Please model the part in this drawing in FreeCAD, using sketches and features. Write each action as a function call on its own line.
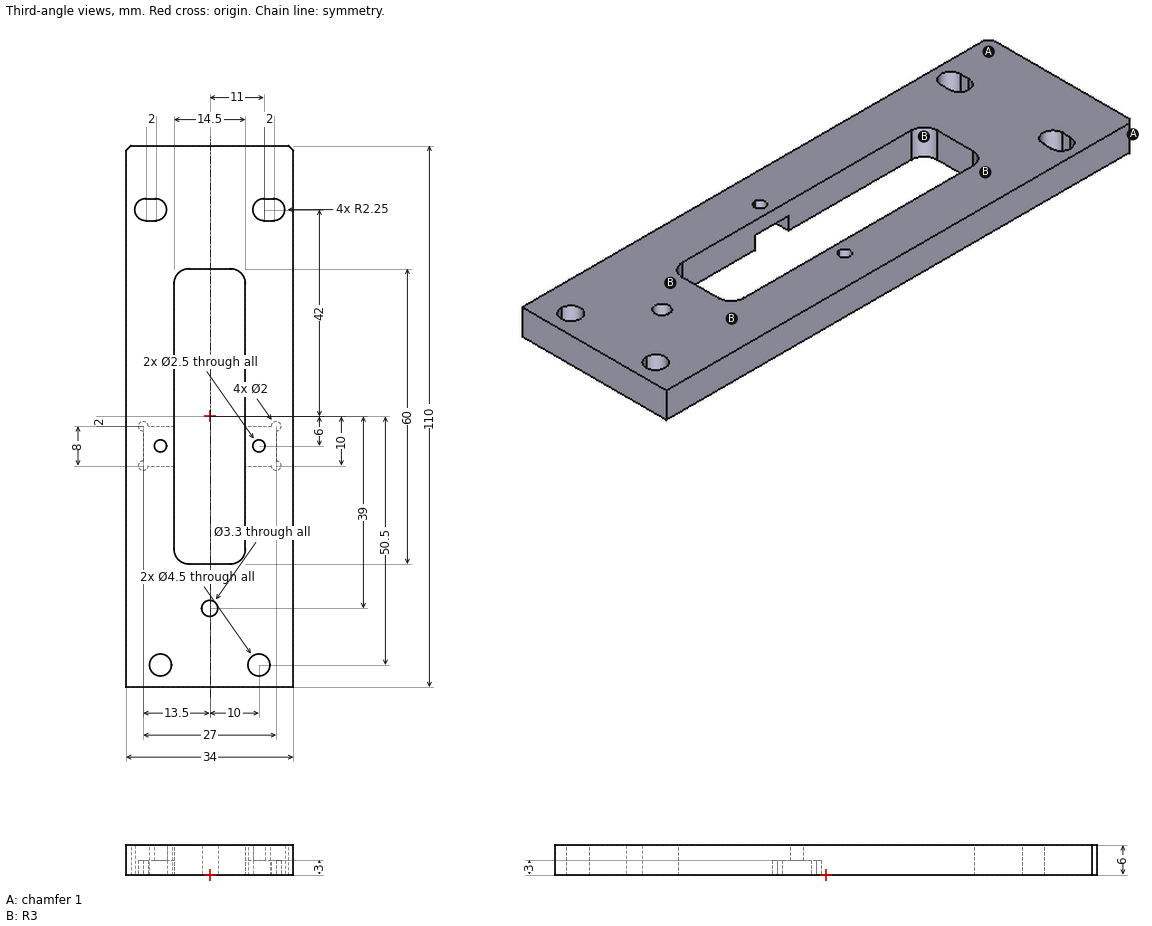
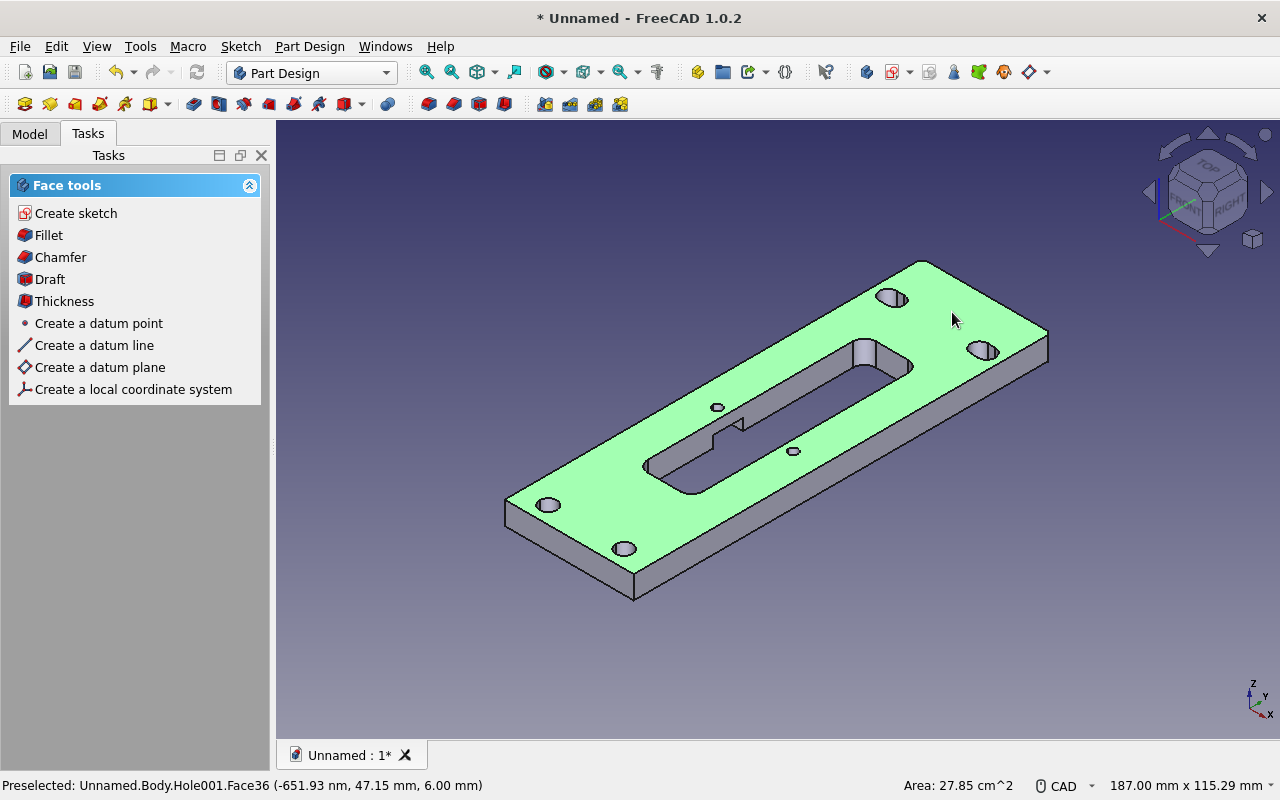
click(892, 72)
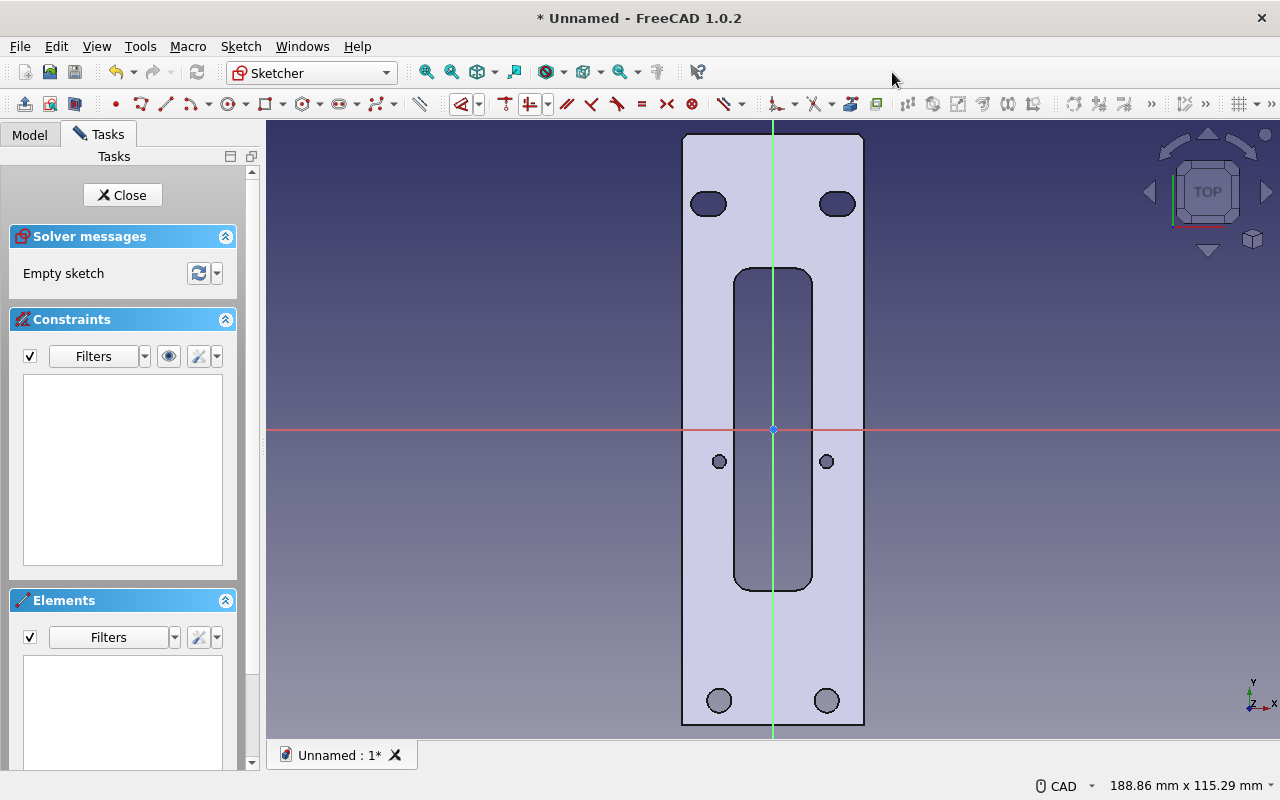
scroll(777, 650, up, 15)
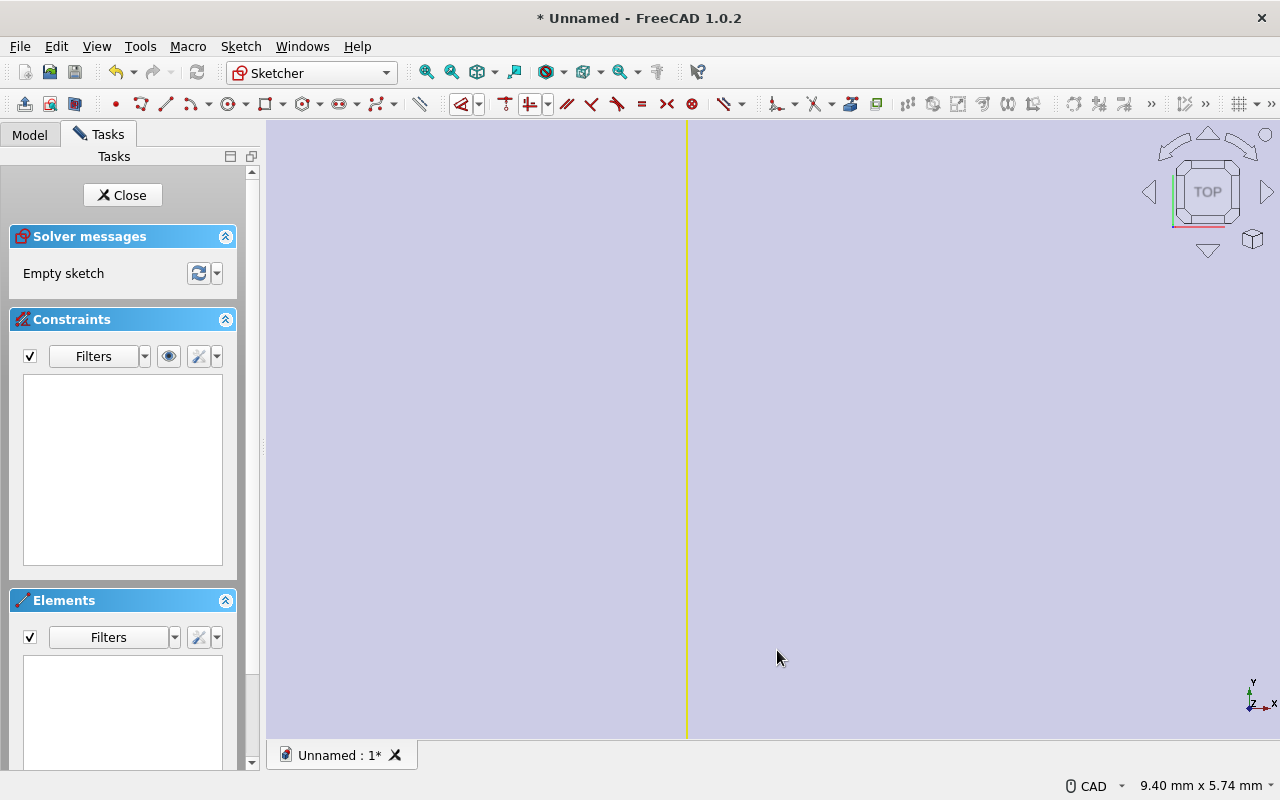
click(228, 104)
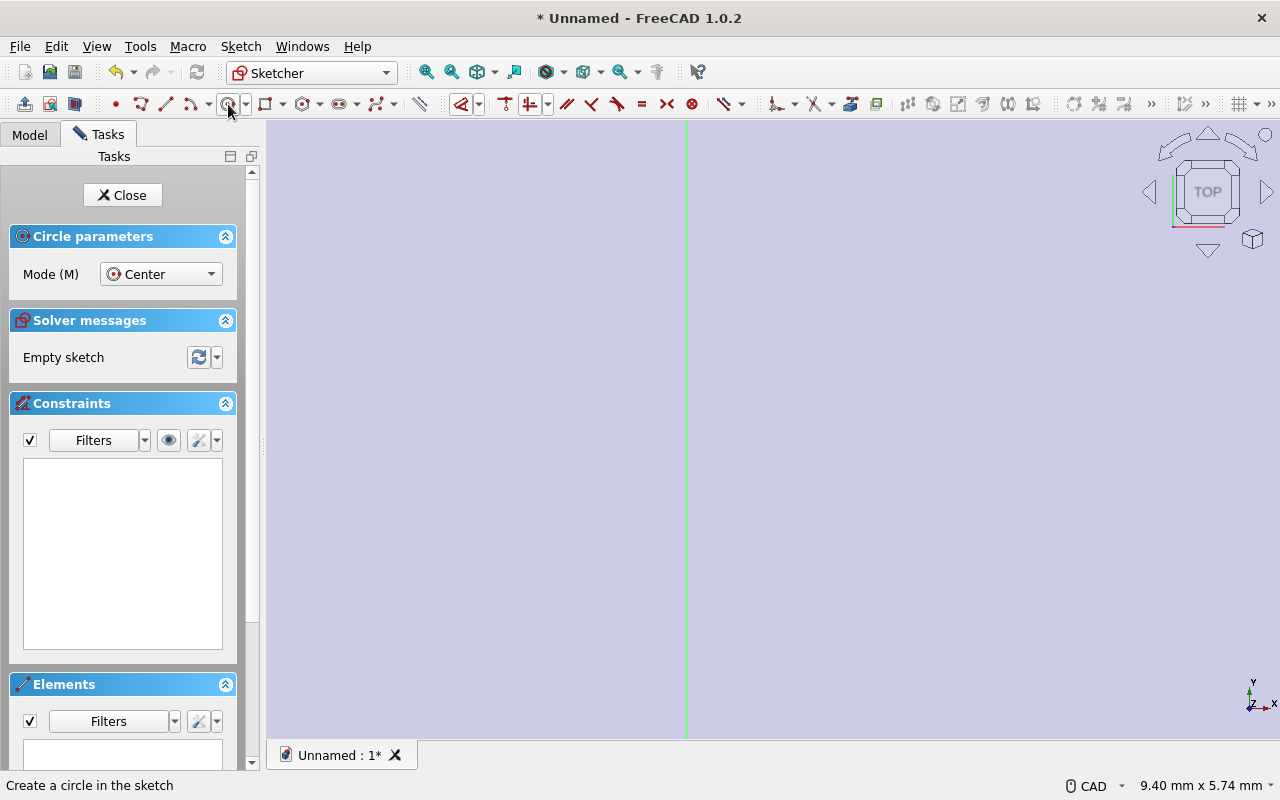
click(687, 411)
click(813, 285)
key(Escape)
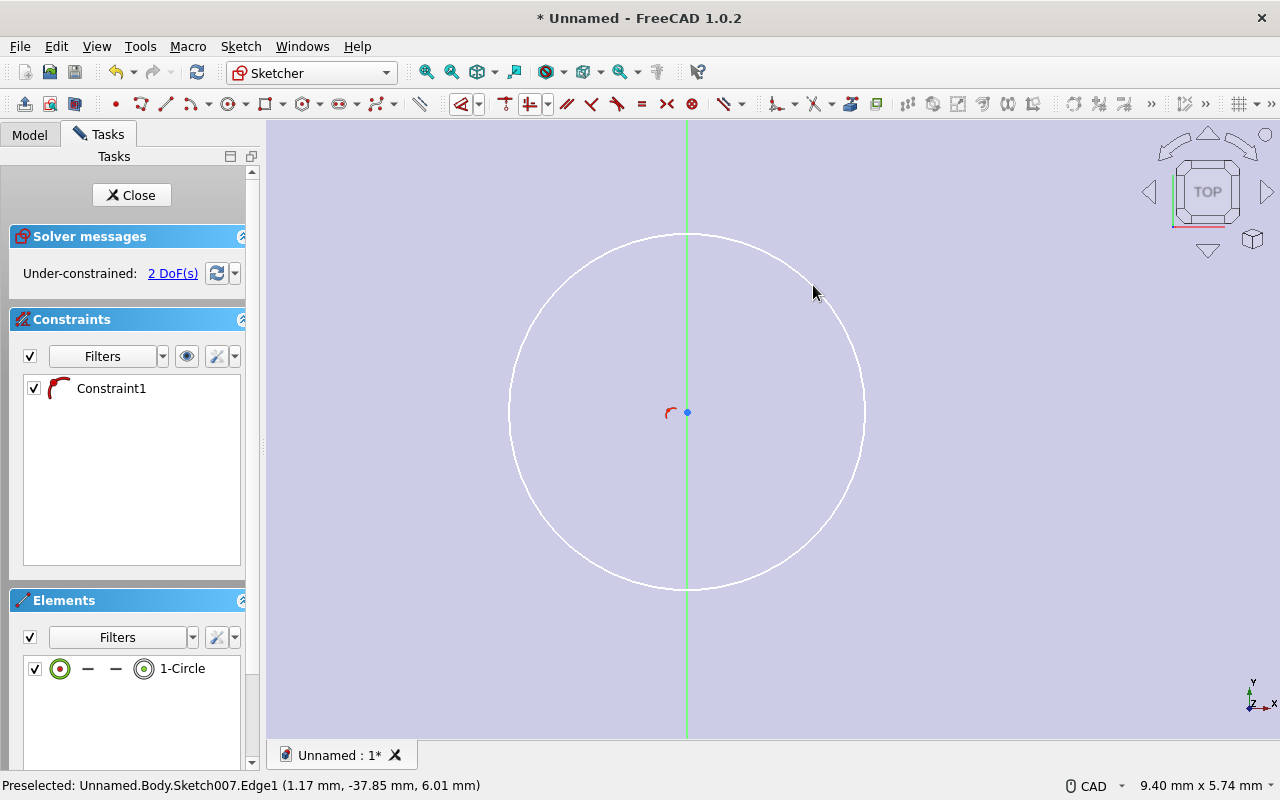
click(813, 286)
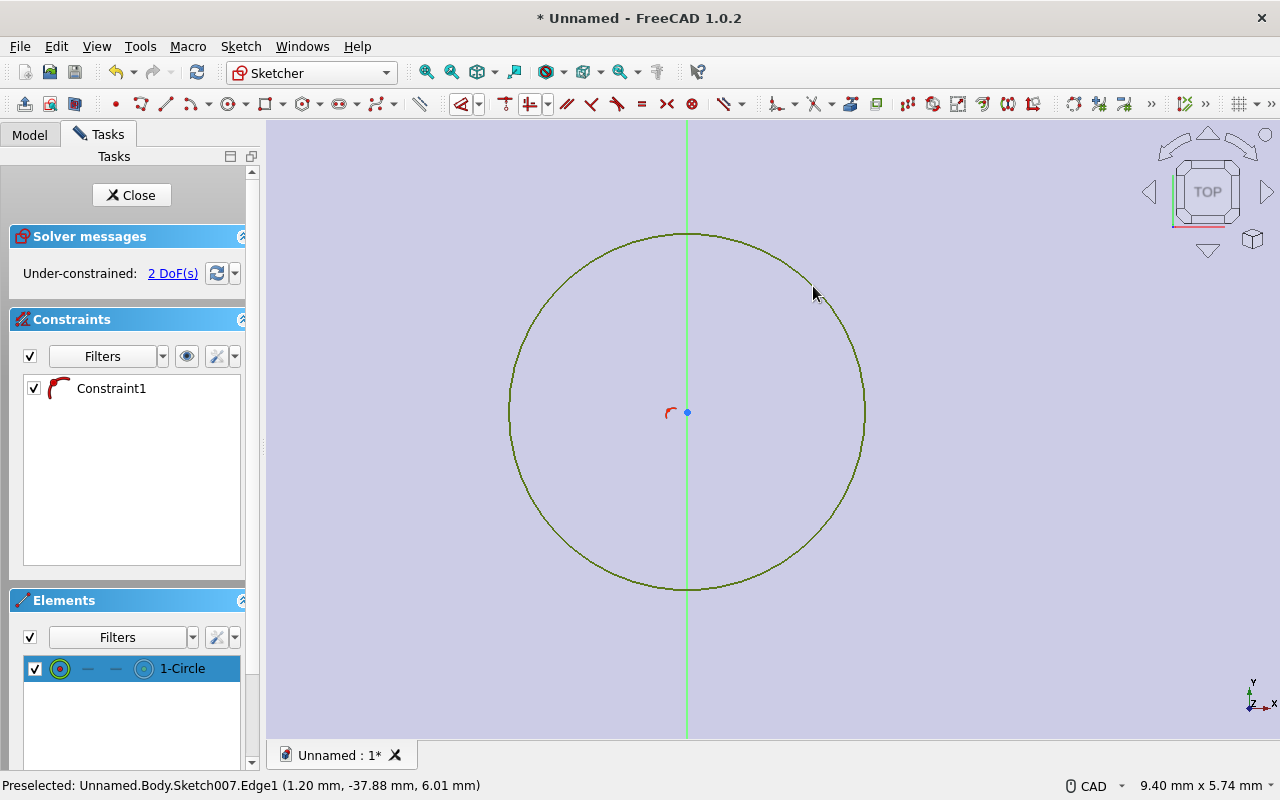
key(k)
key(o)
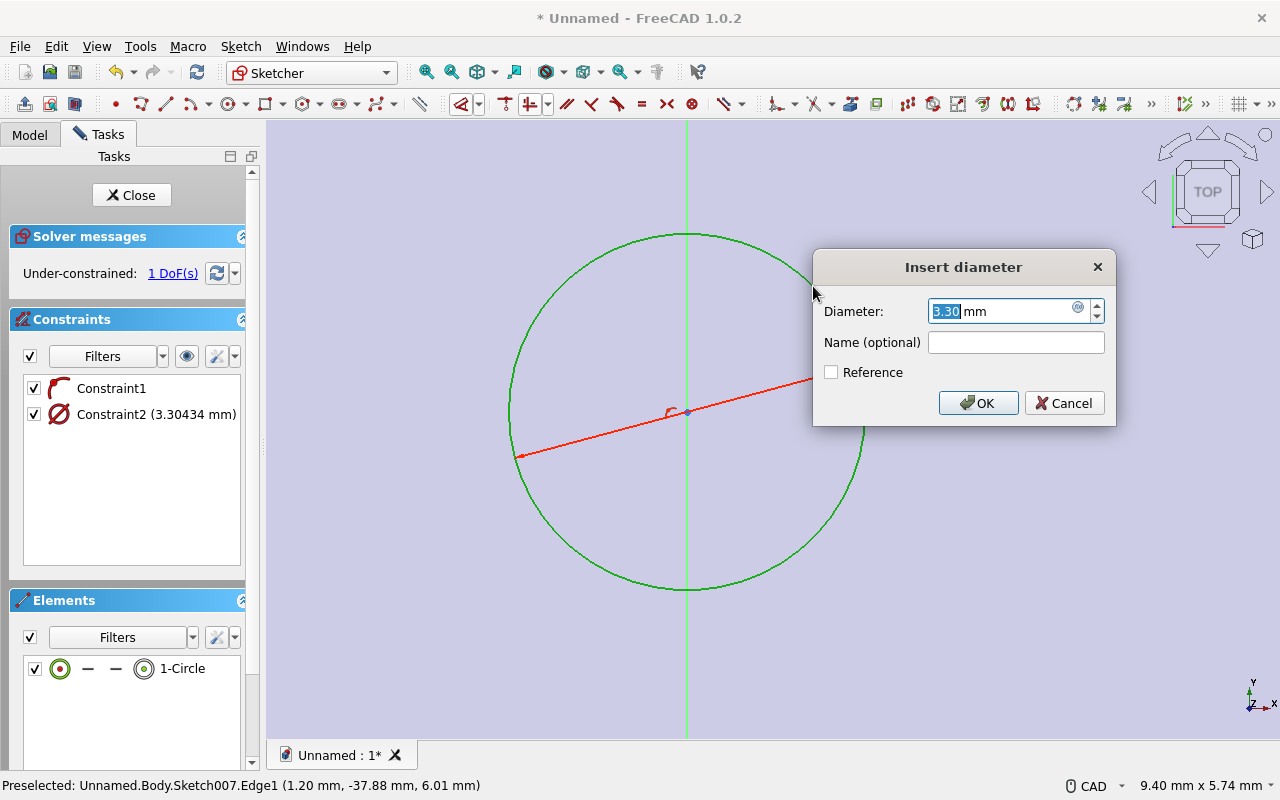
text(3.3)
key(Return)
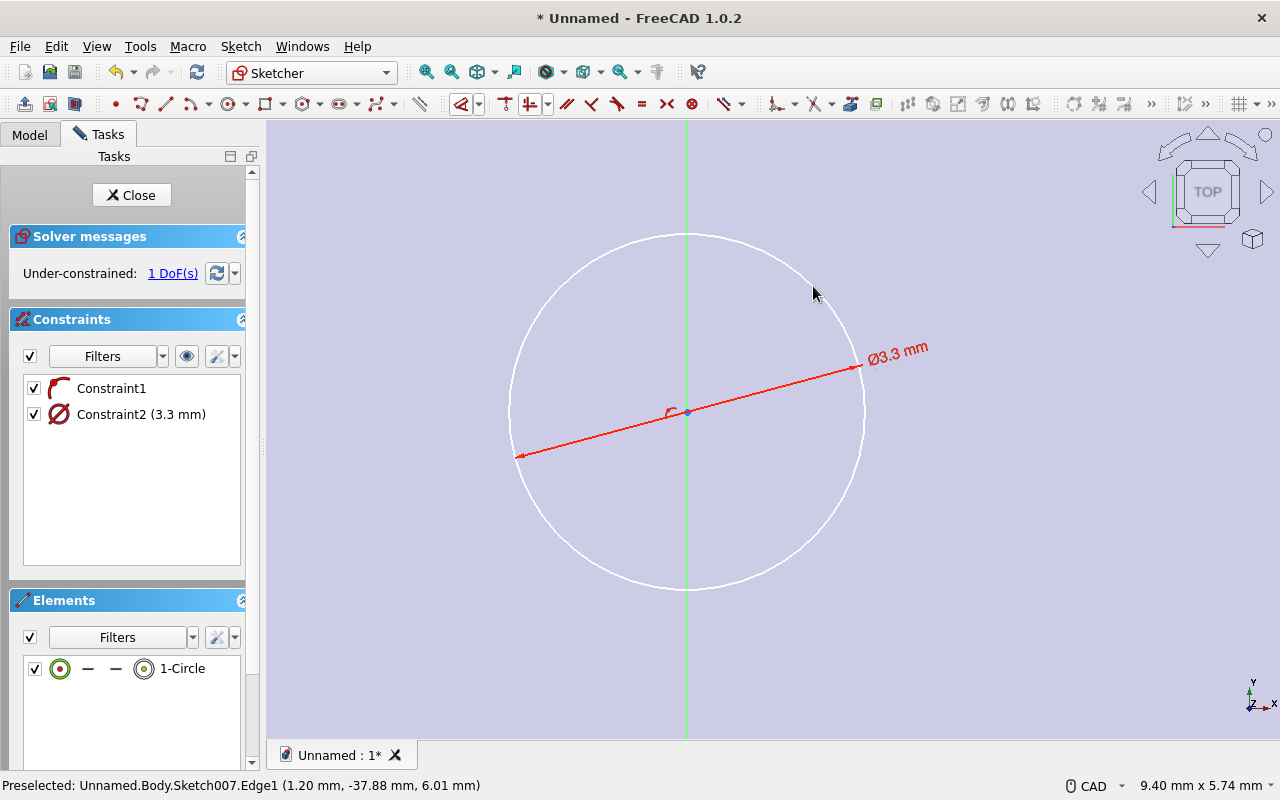
click(687, 412)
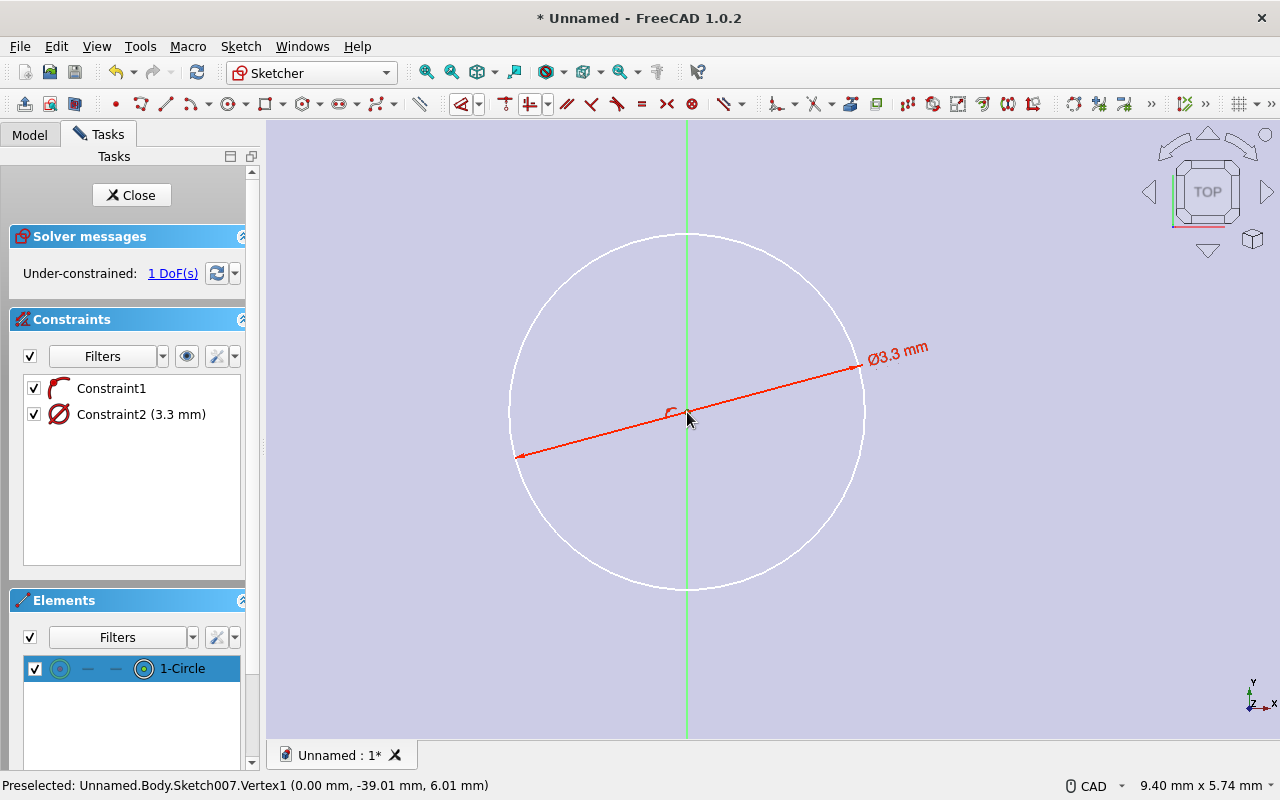
key(i)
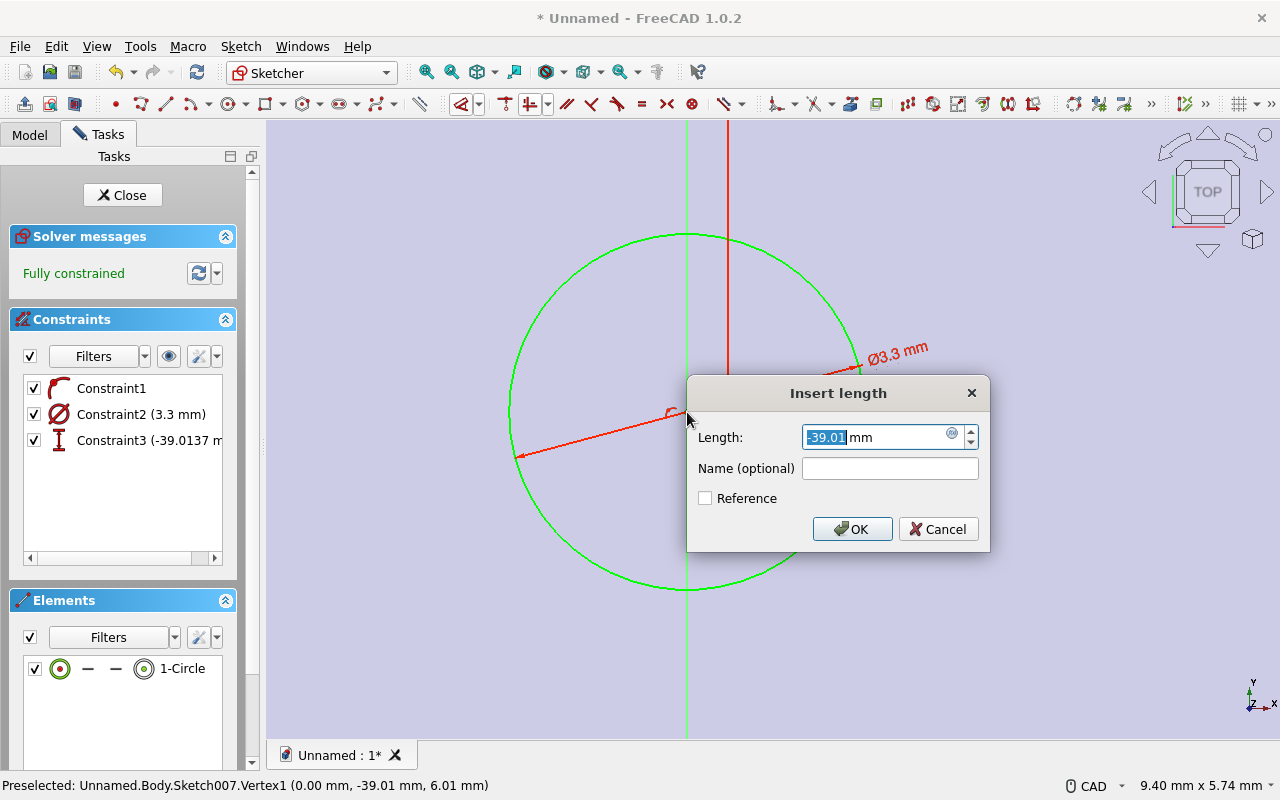
text(-39)
key(Return)